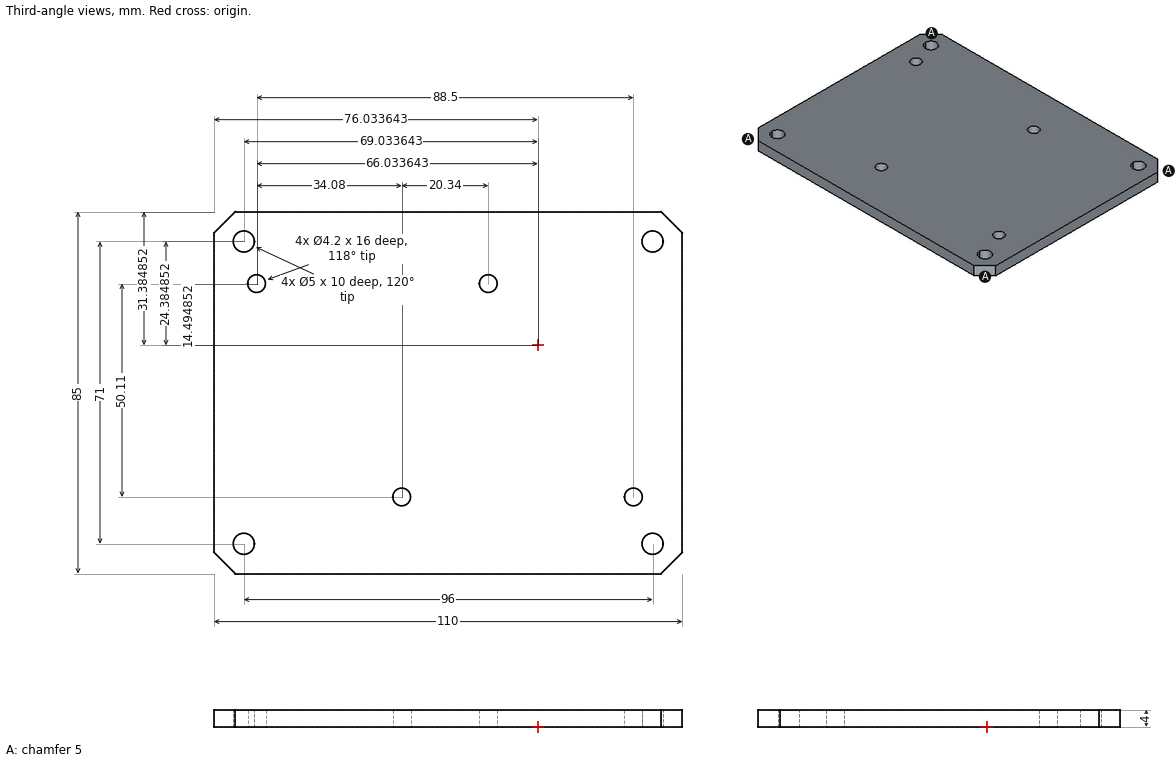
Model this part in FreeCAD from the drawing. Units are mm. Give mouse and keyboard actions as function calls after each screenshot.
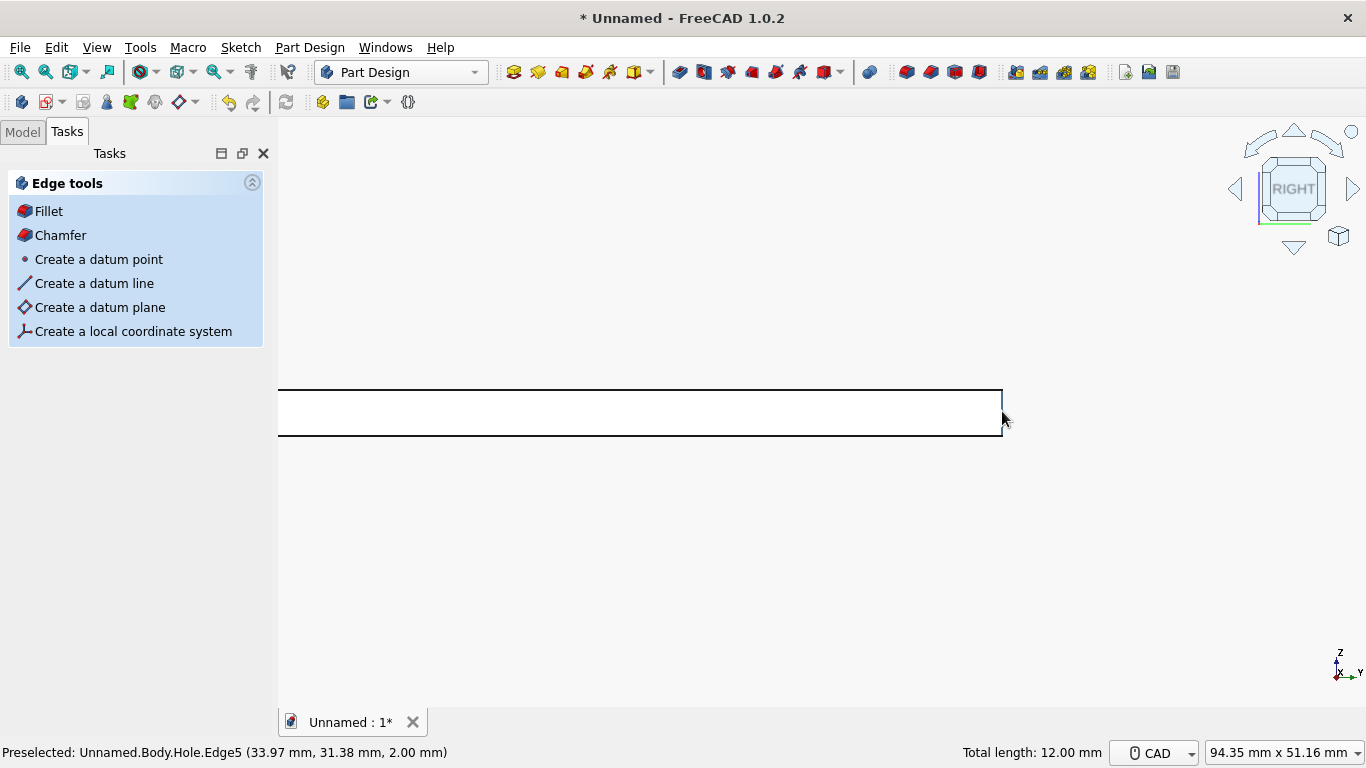
click(22, 72)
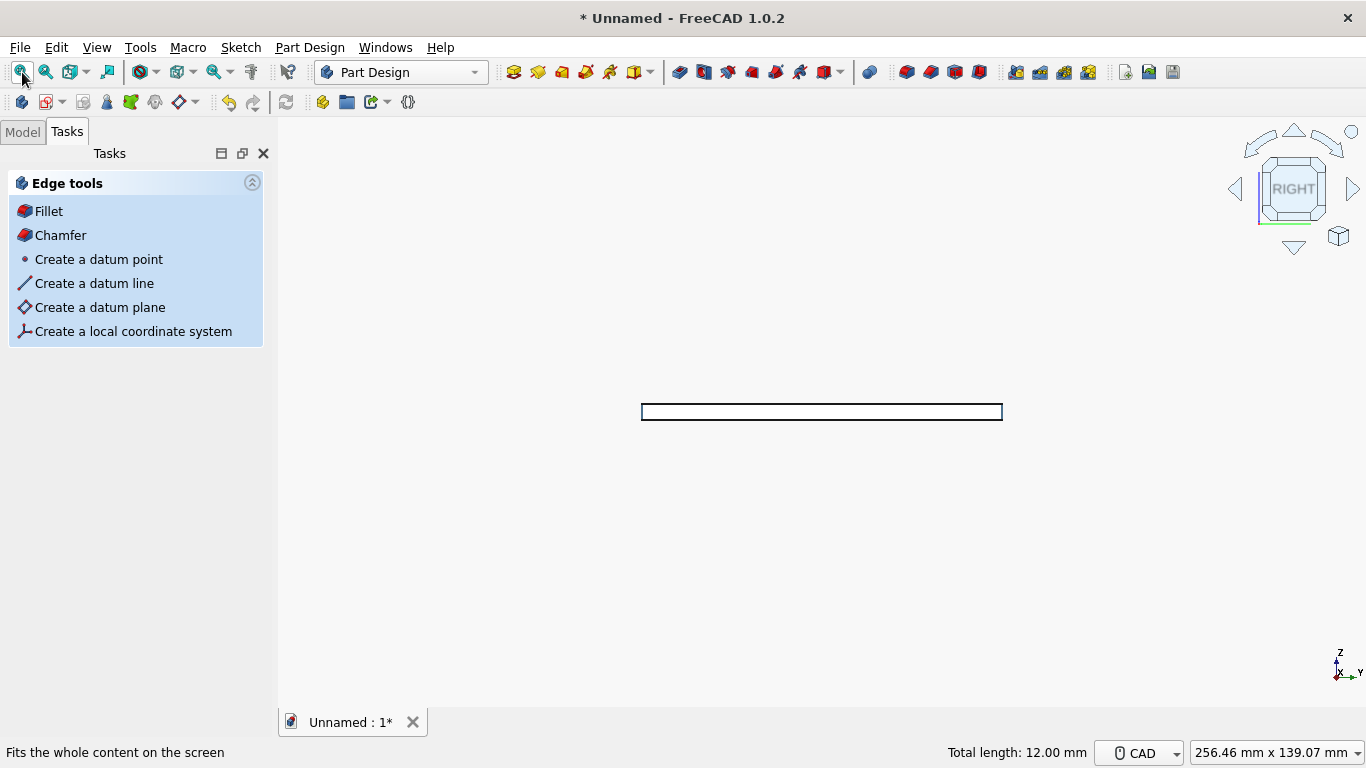
key(5)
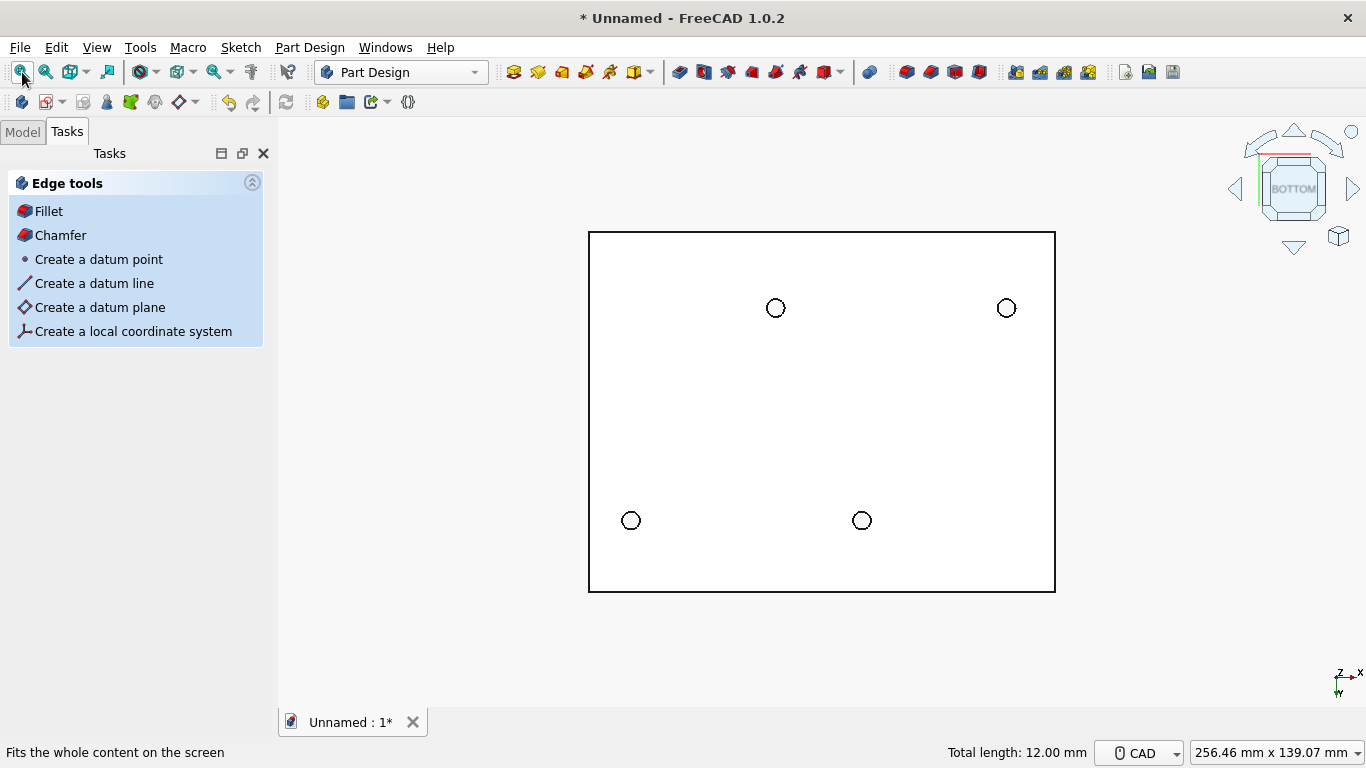
scroll(589, 591, up, 5)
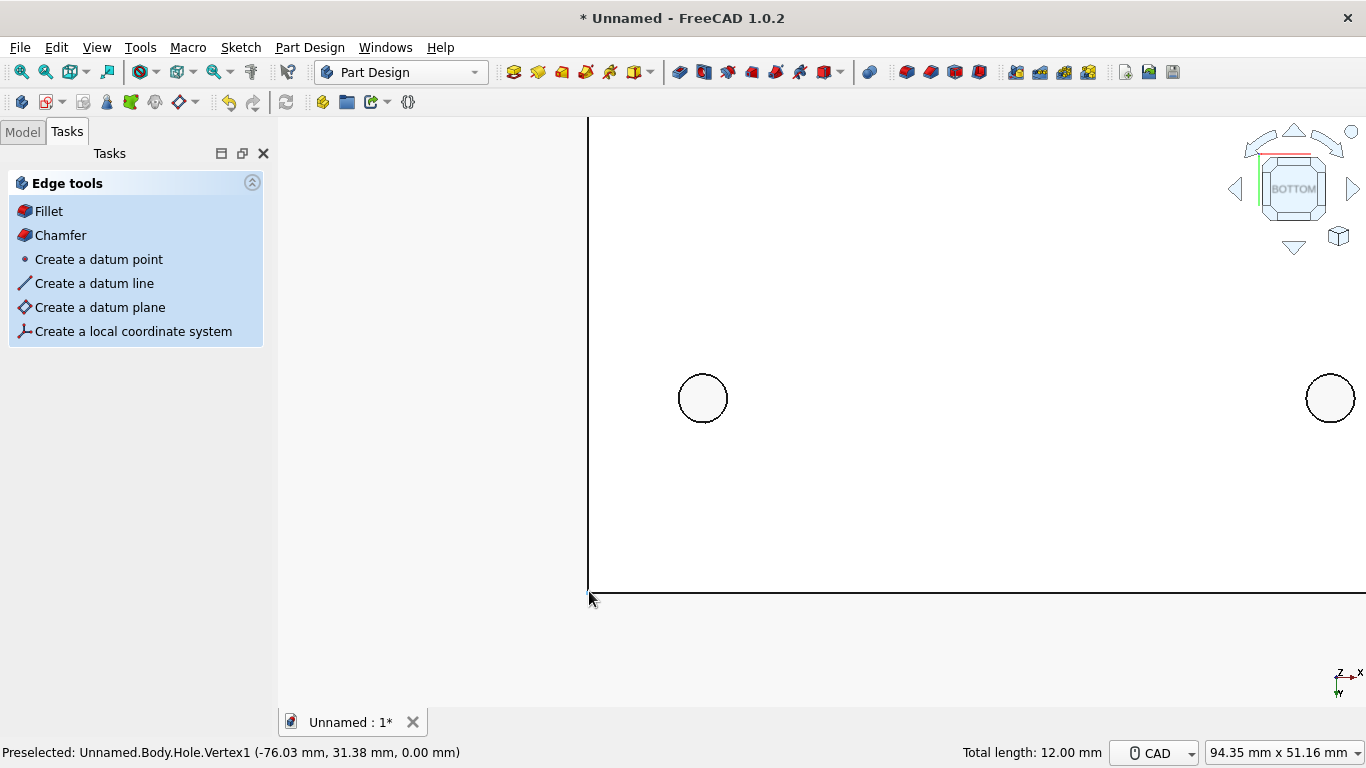
click(22, 72)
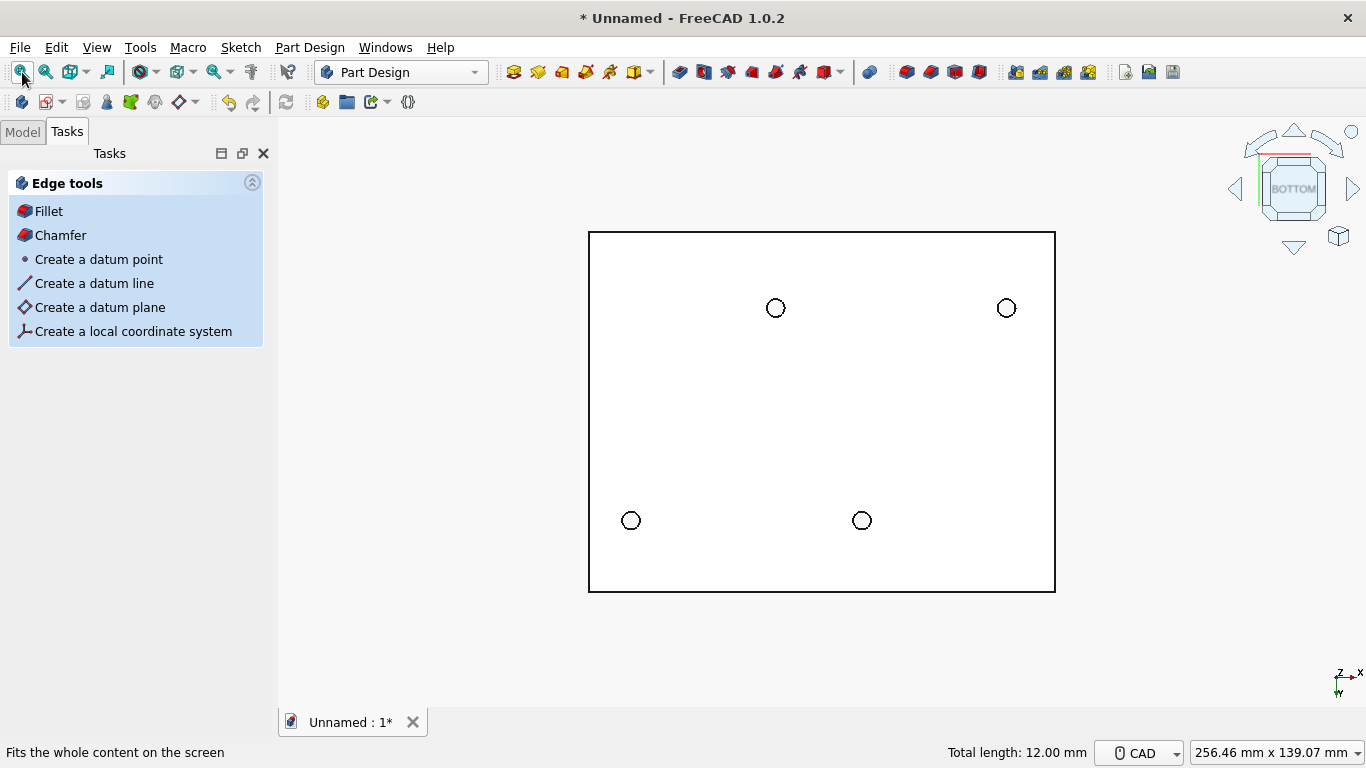
key(4)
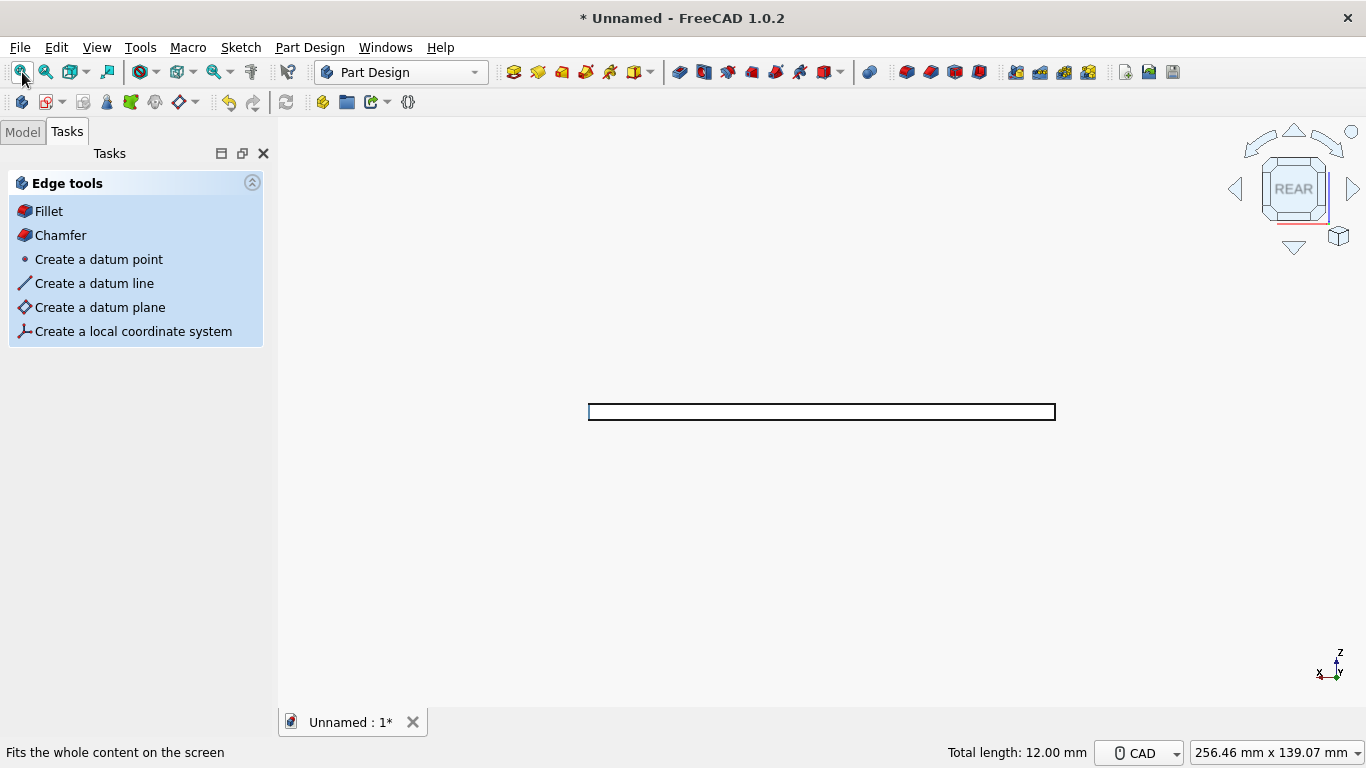
click(22, 72)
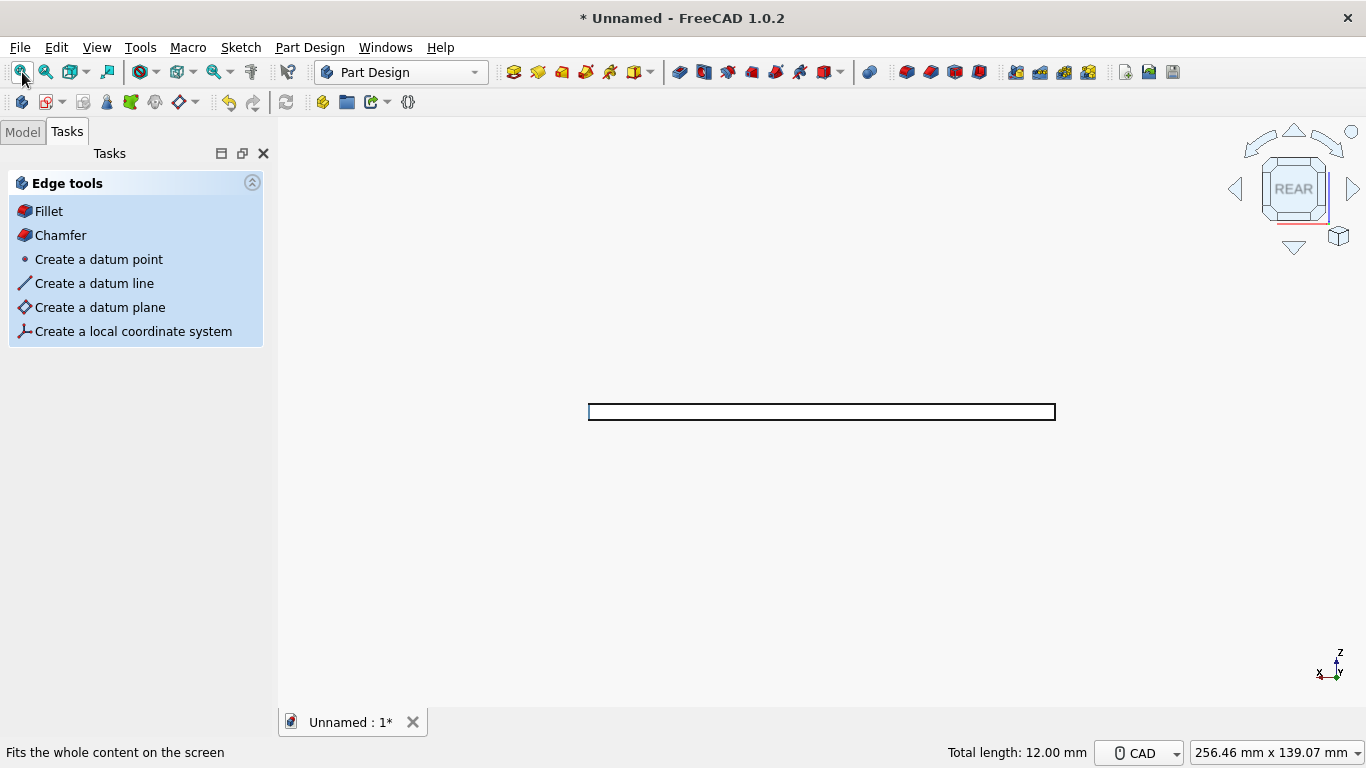
click(1055, 411, ctrl)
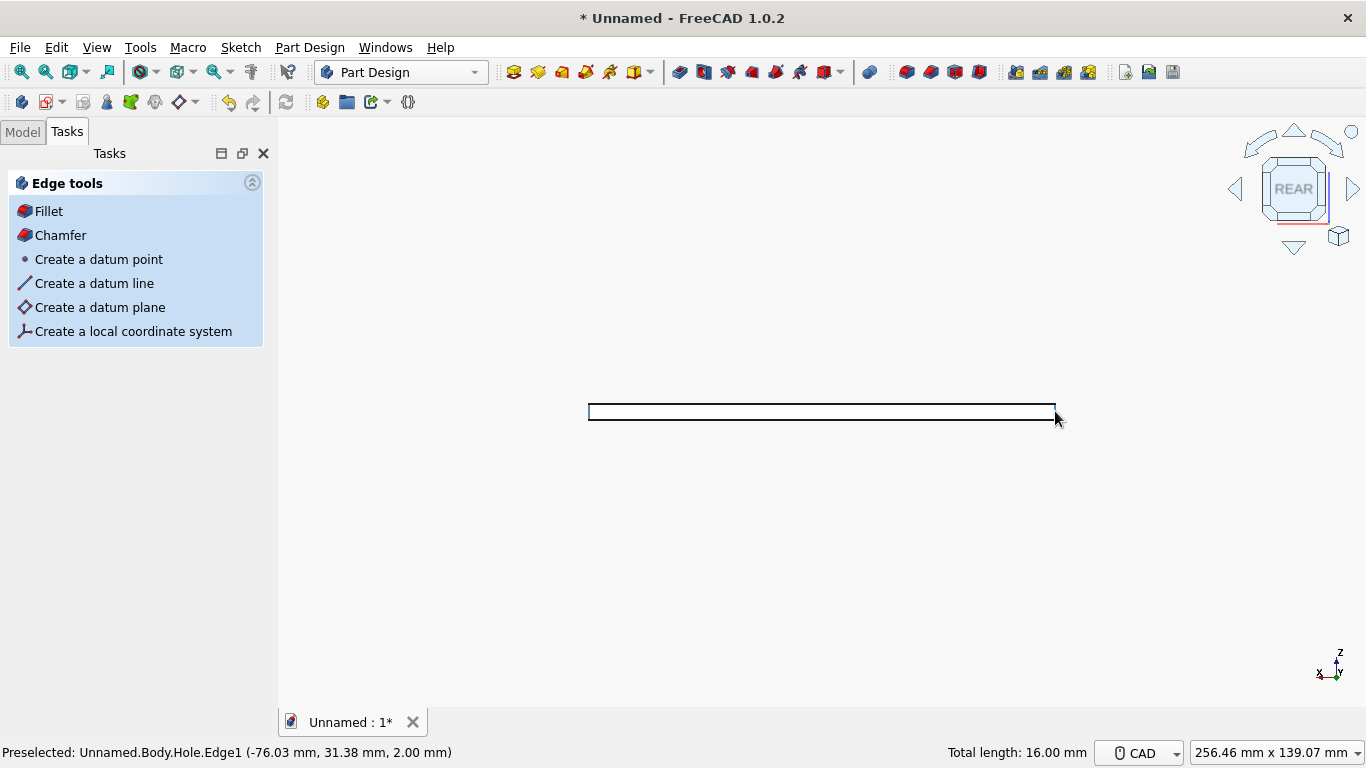
click(932, 72)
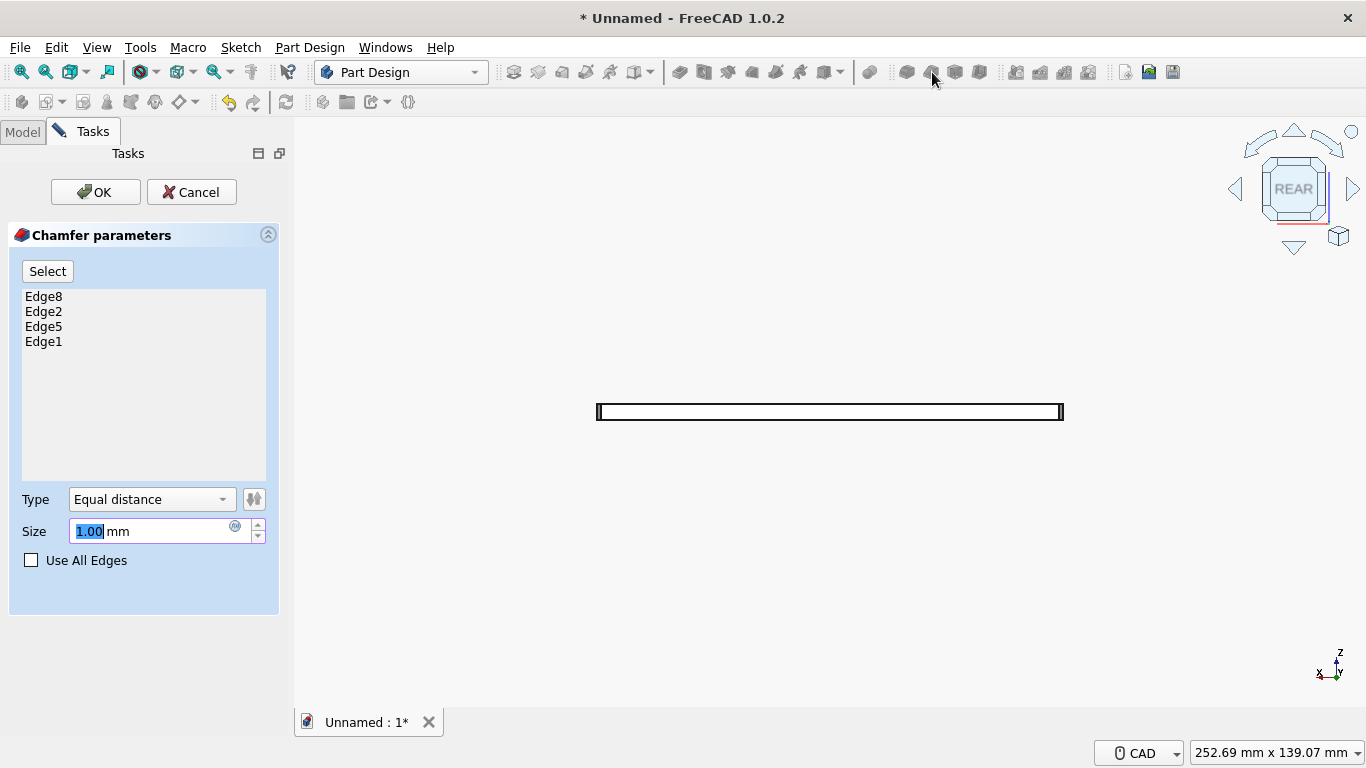
text(5)
key(Tab)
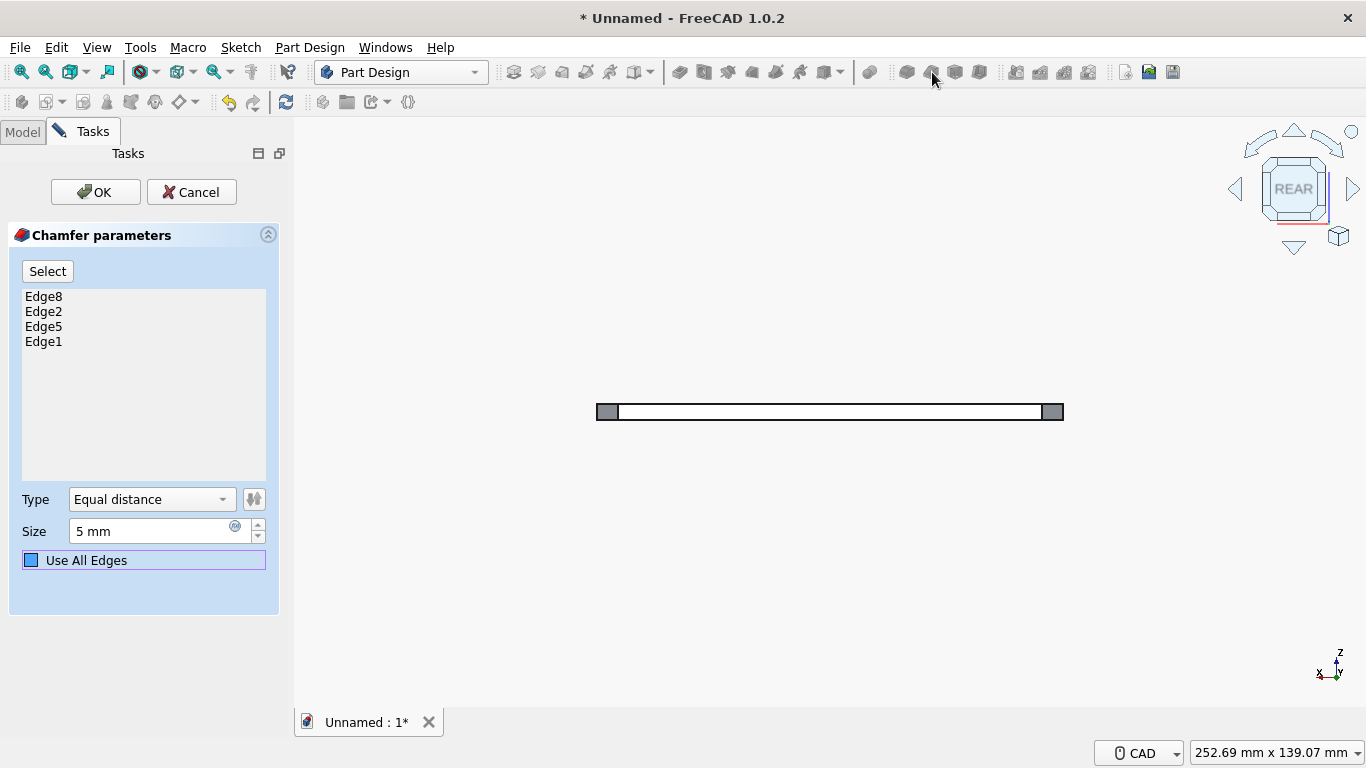
click(96, 192)